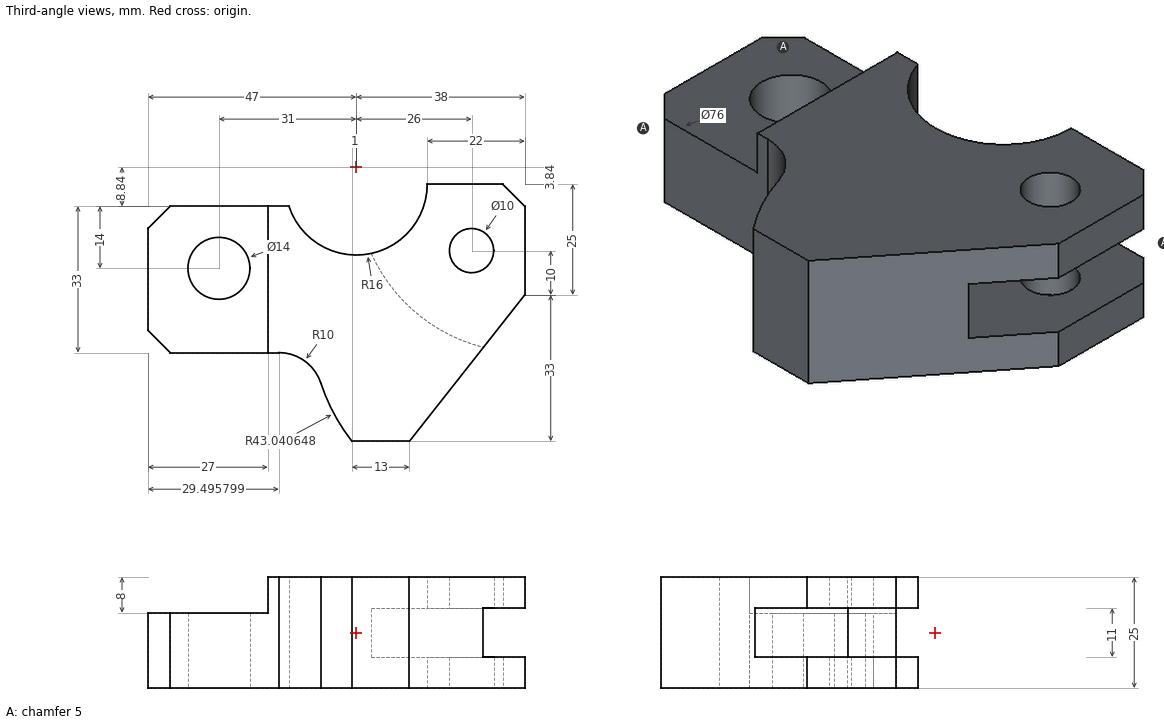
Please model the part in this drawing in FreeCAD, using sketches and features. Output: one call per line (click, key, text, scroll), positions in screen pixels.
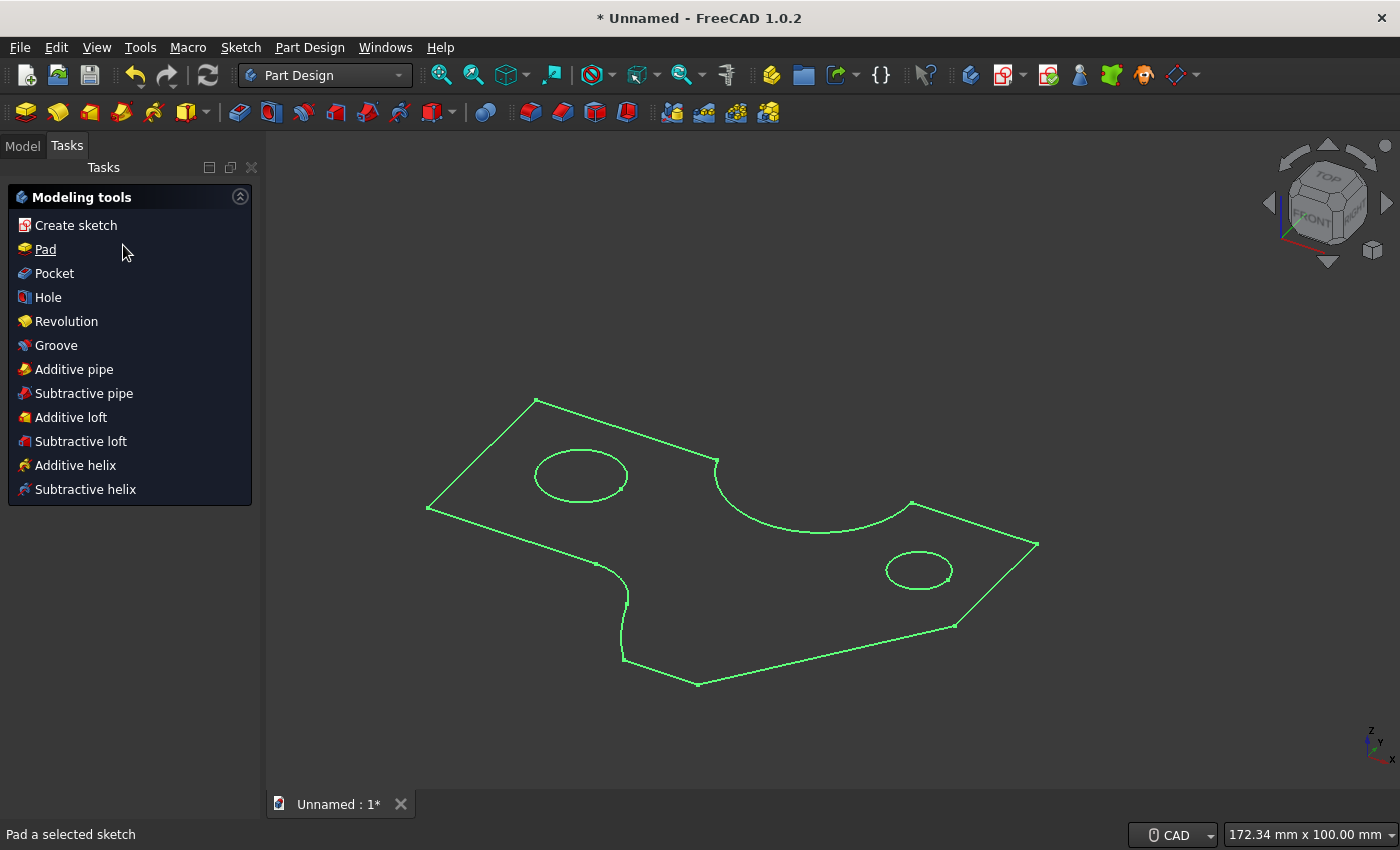
click(26, 112)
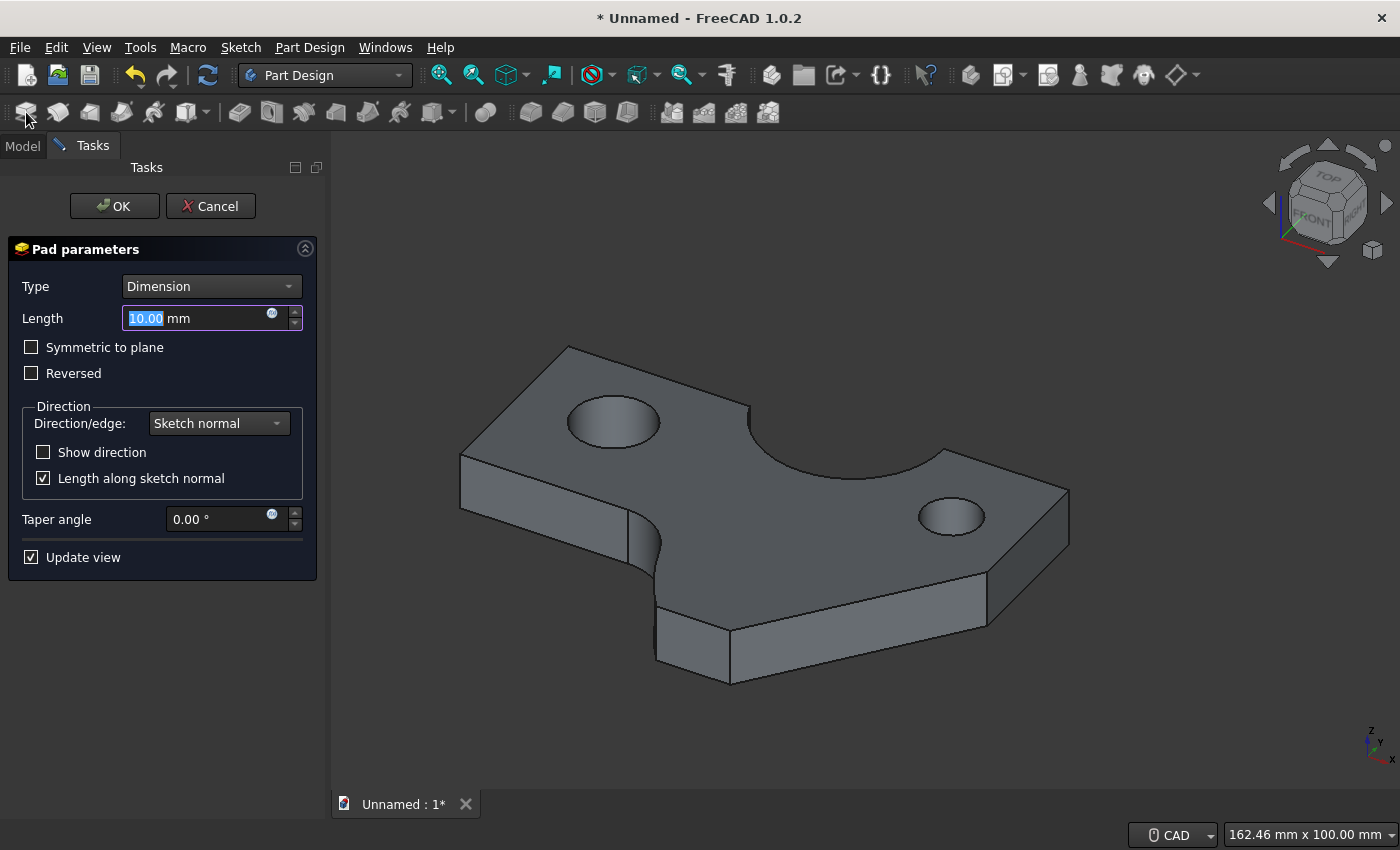
text(25)
key(Tab)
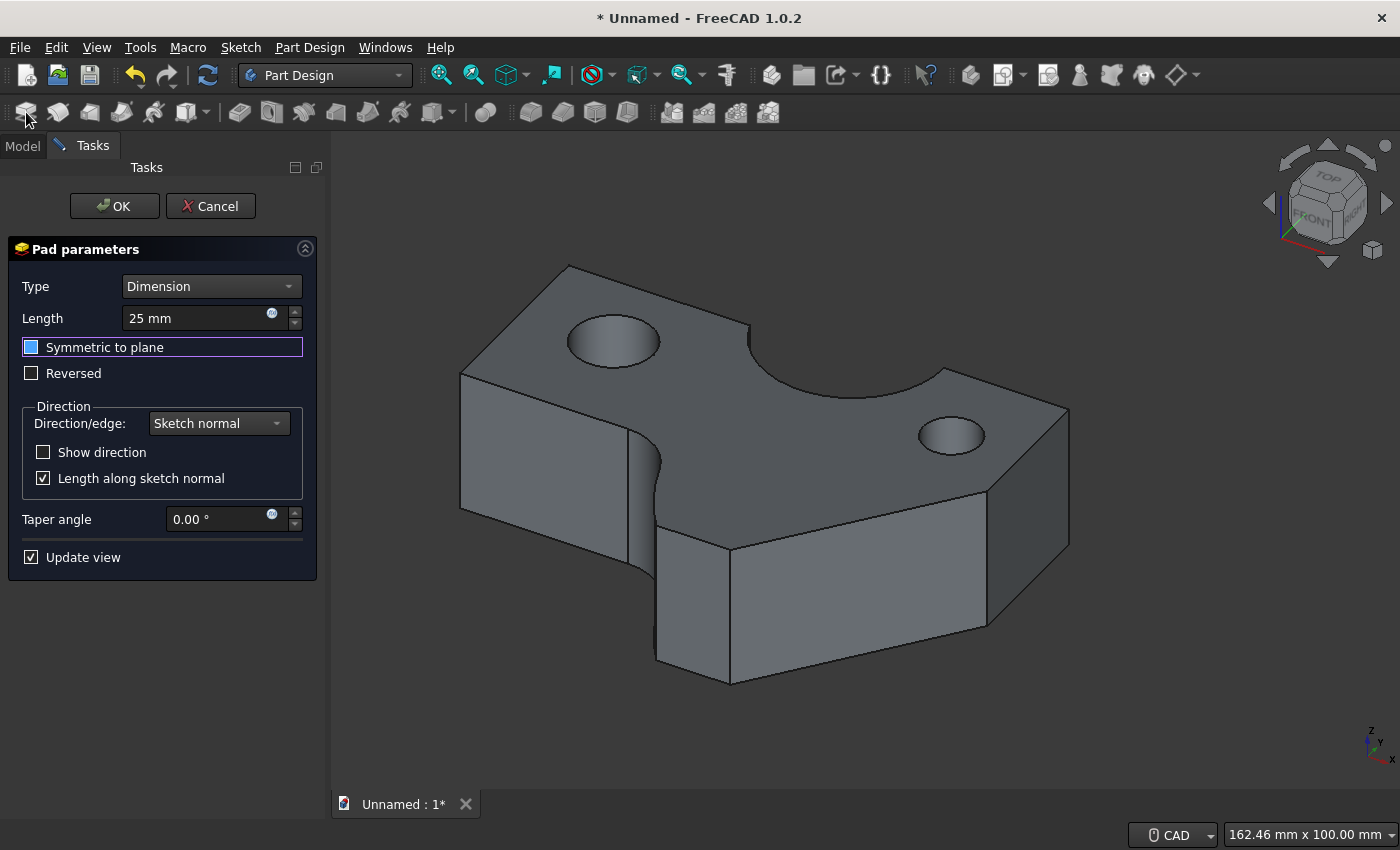
click(30, 347)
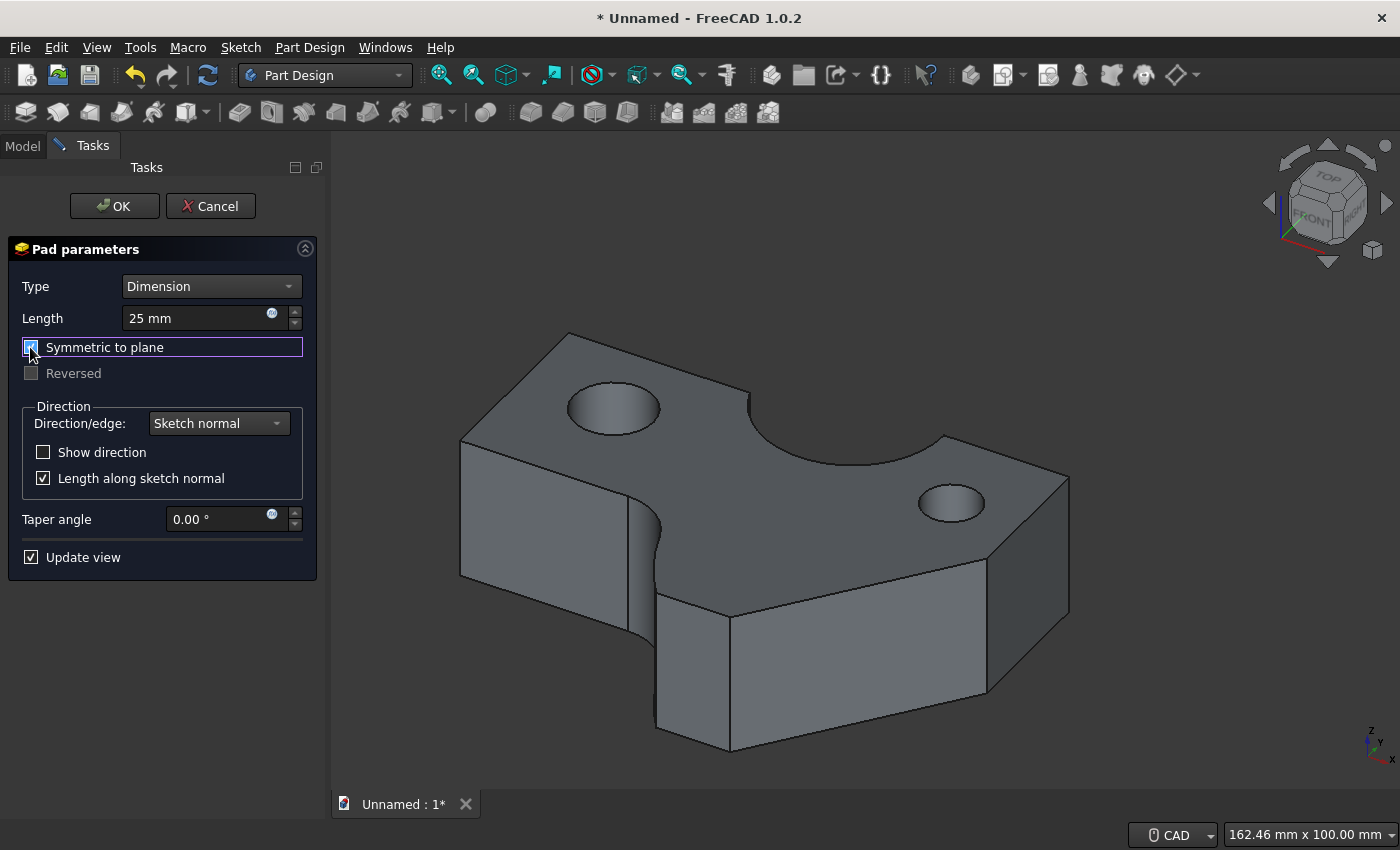
click(115, 206)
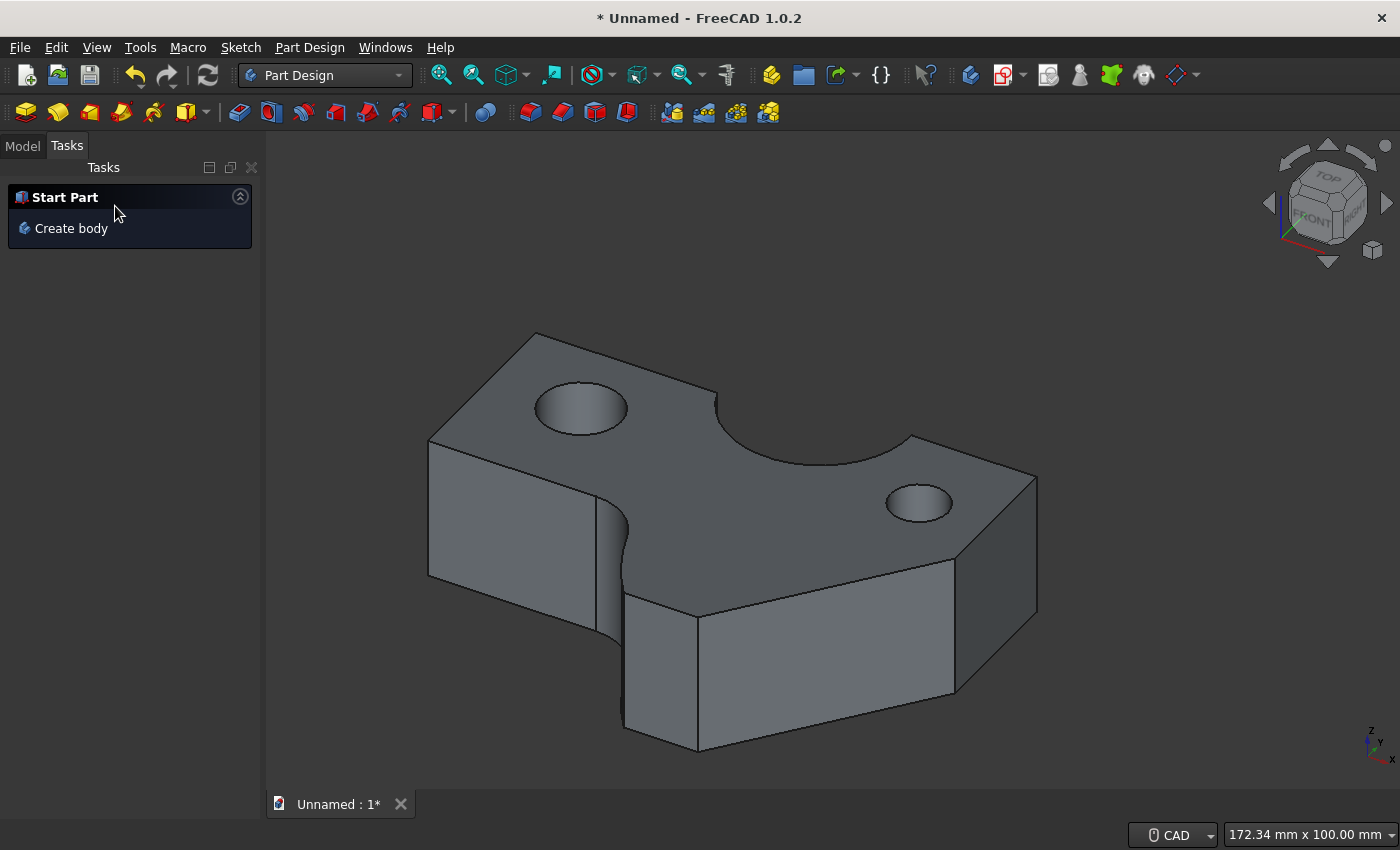
key(v)
key(f)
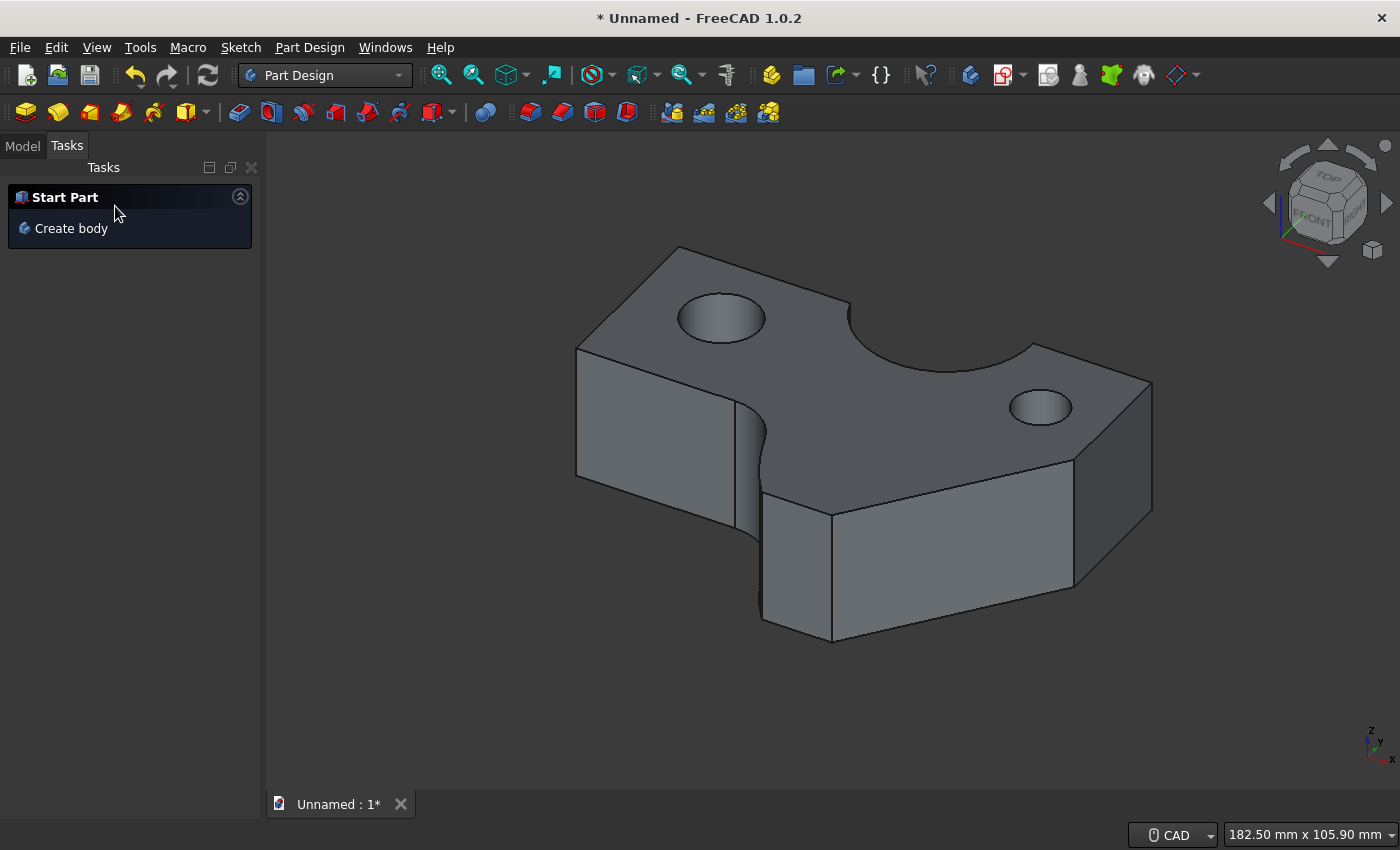
key(0)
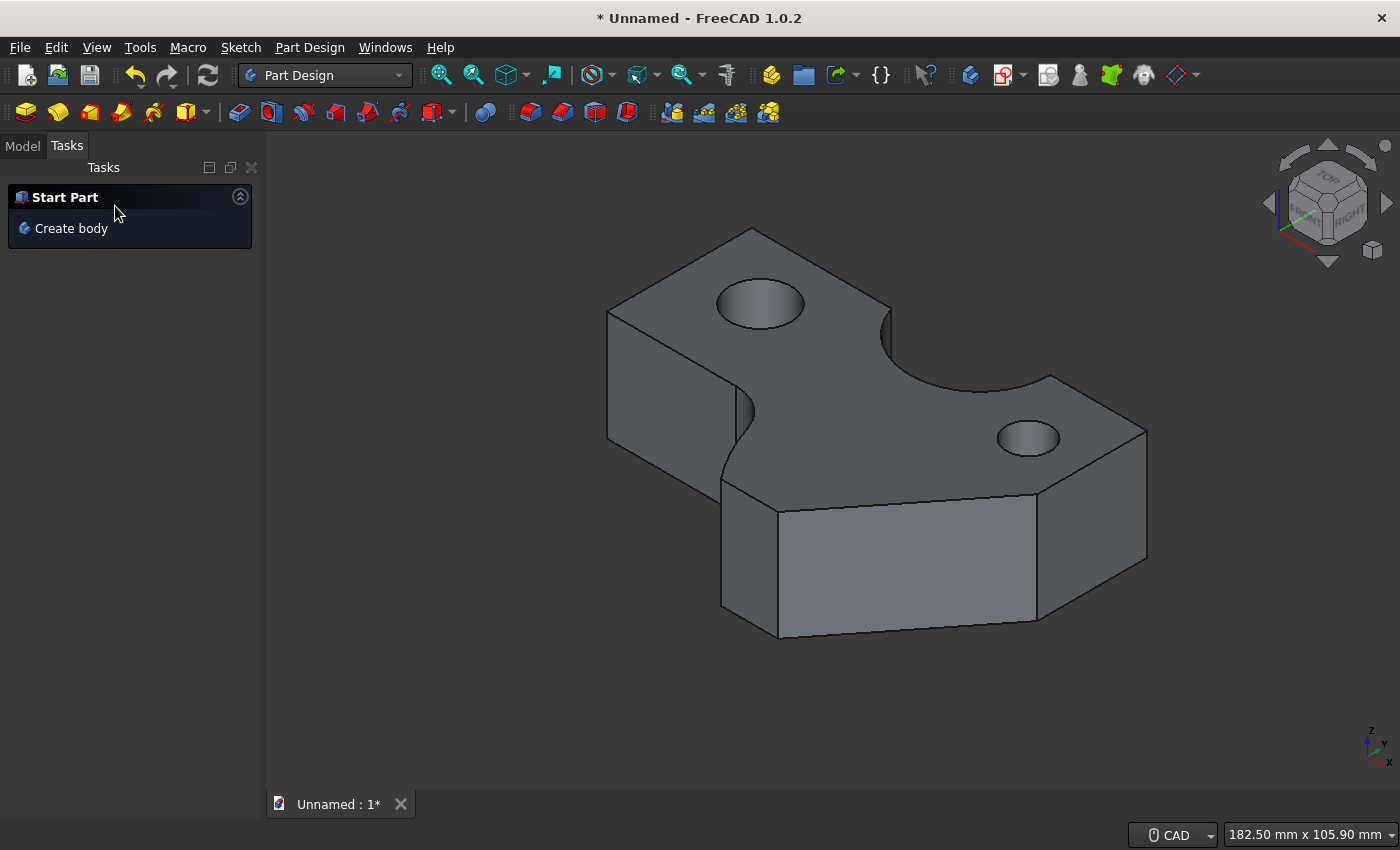
key(2)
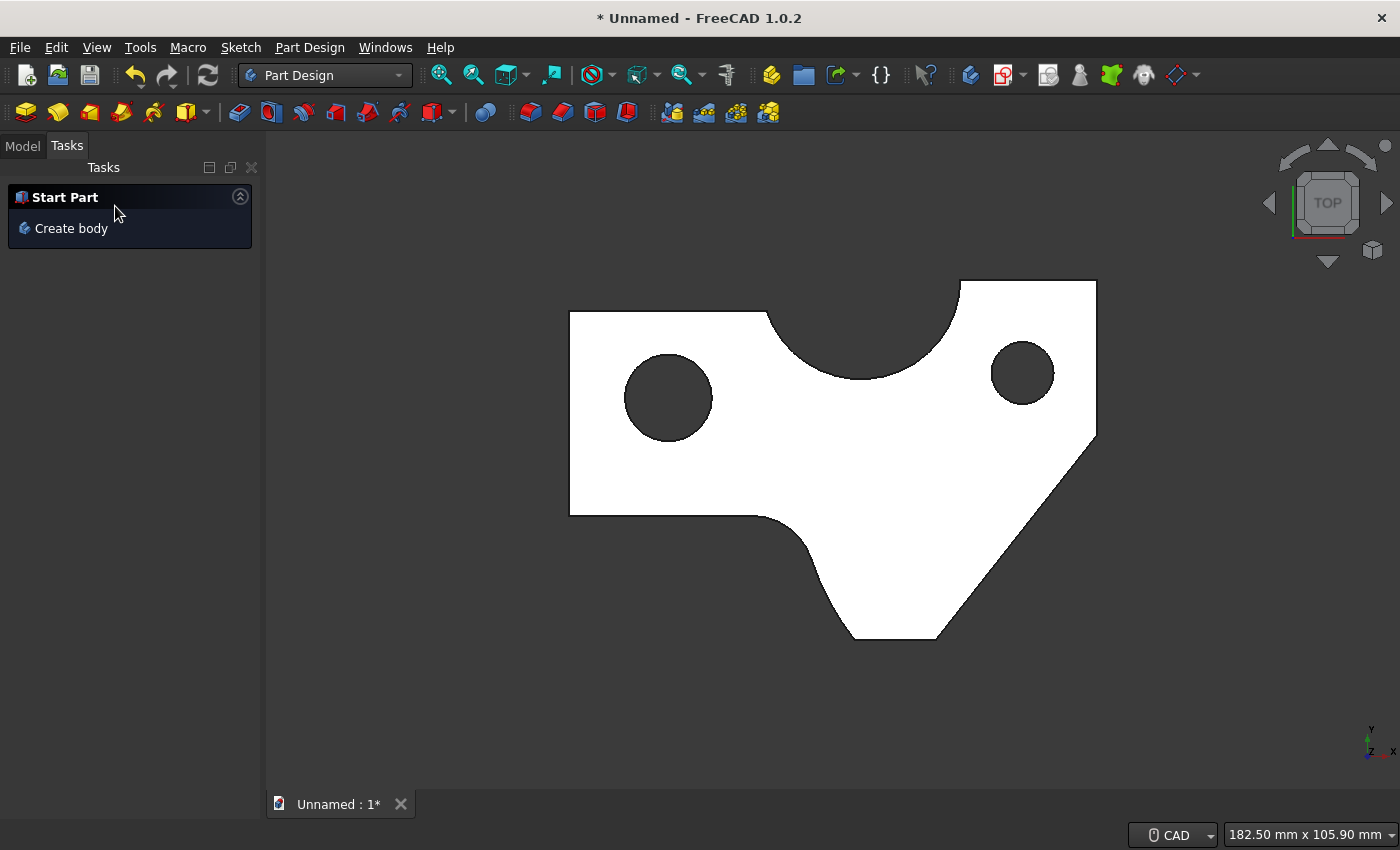
key(1)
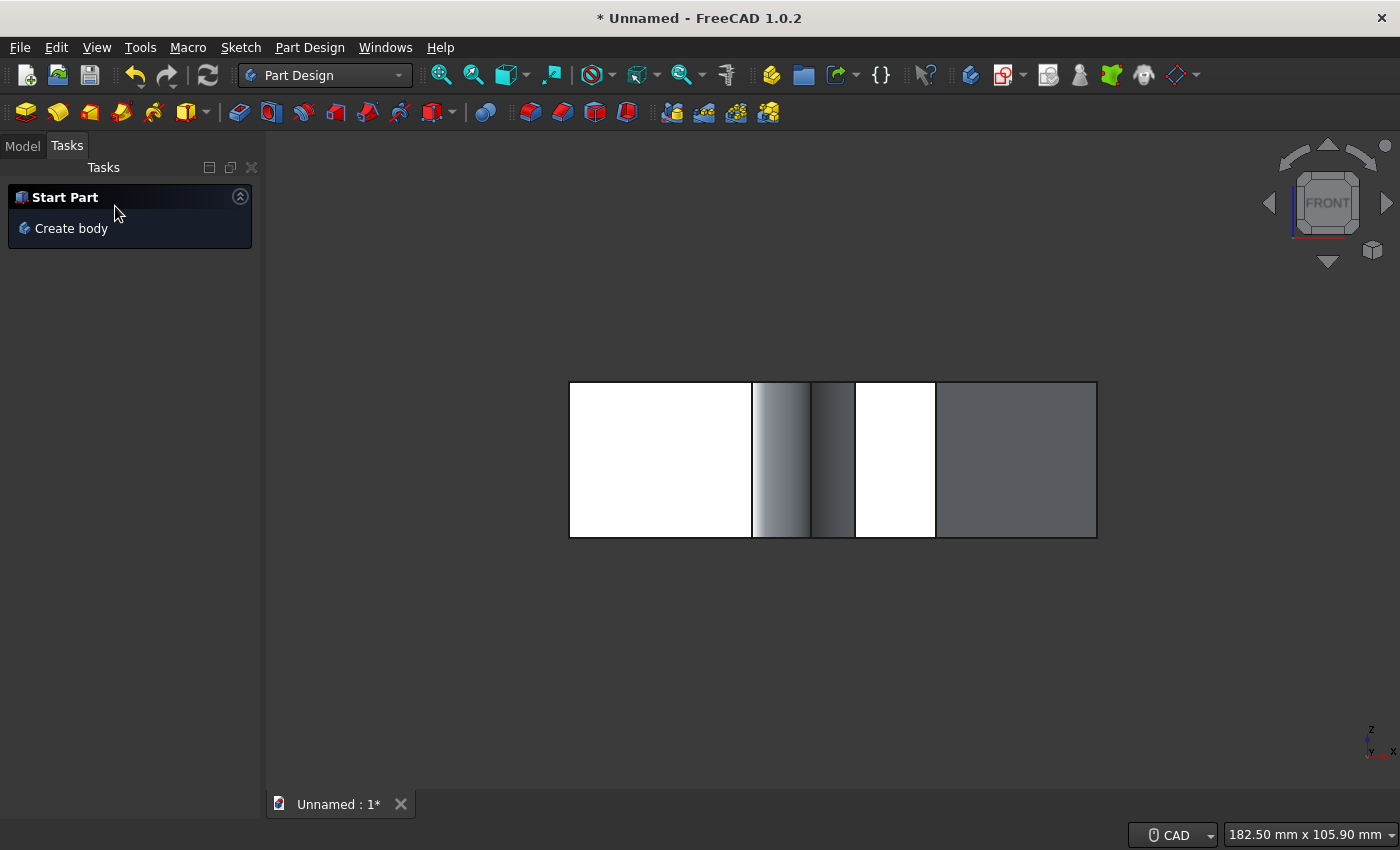
click(569, 459)